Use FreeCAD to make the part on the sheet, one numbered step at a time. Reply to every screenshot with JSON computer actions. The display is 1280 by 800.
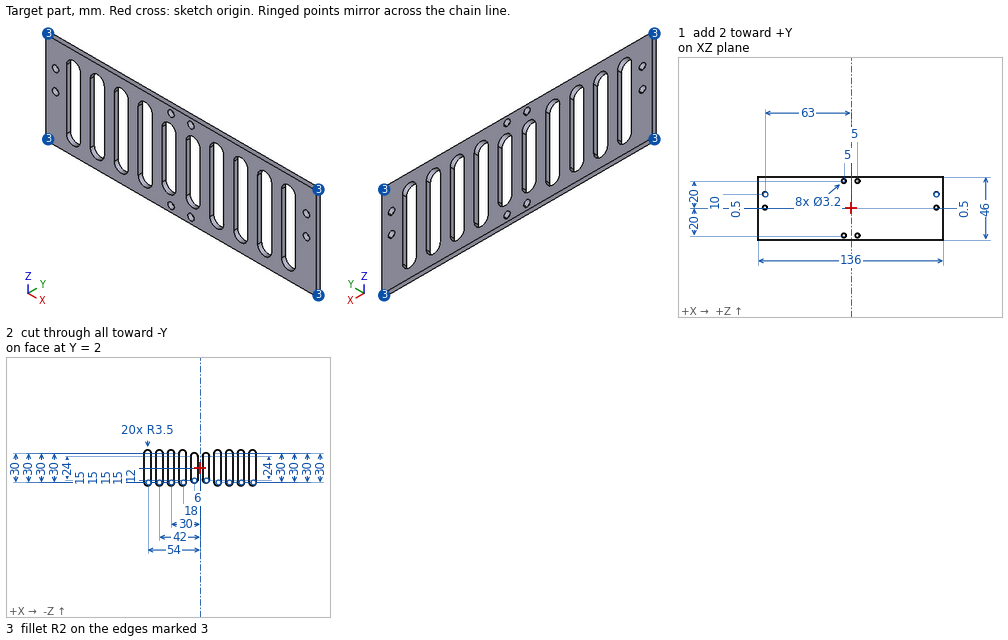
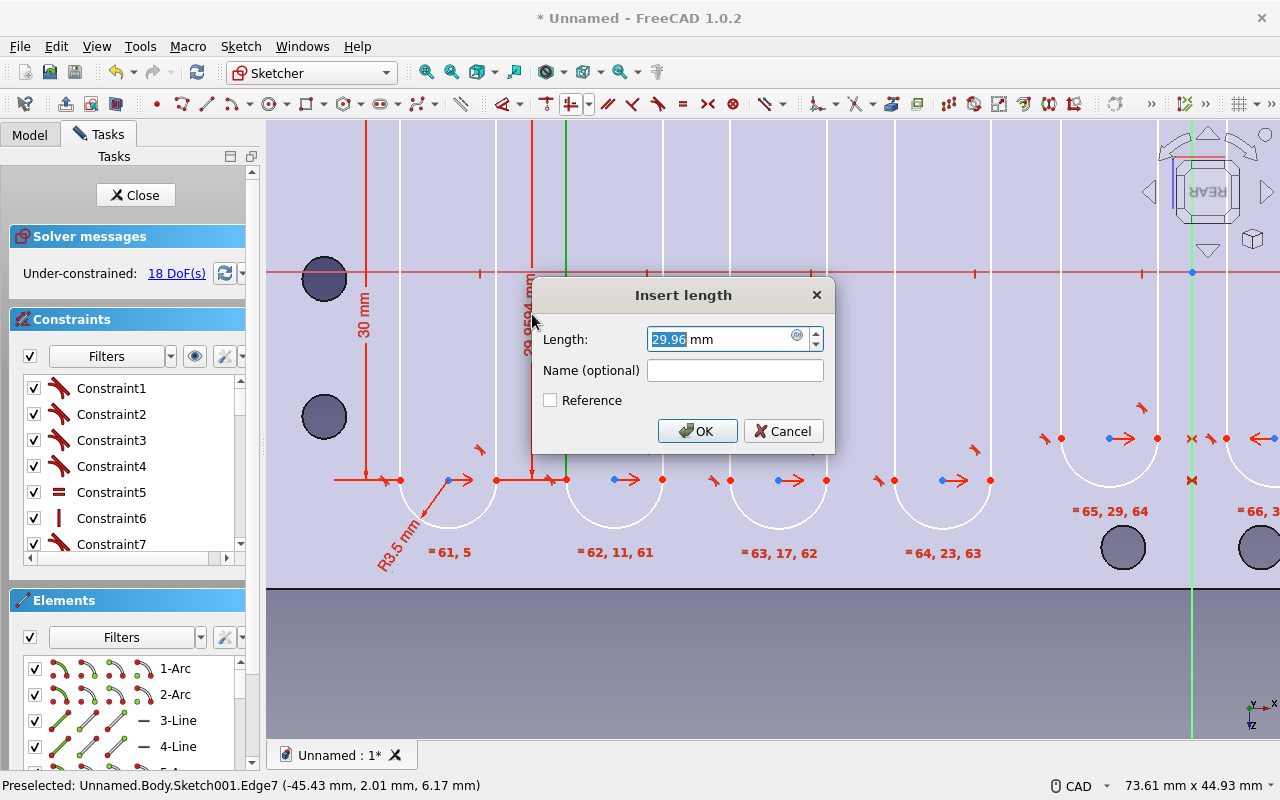
{"action": "type", "text": "30"}
{"action": "key", "text": "Return"}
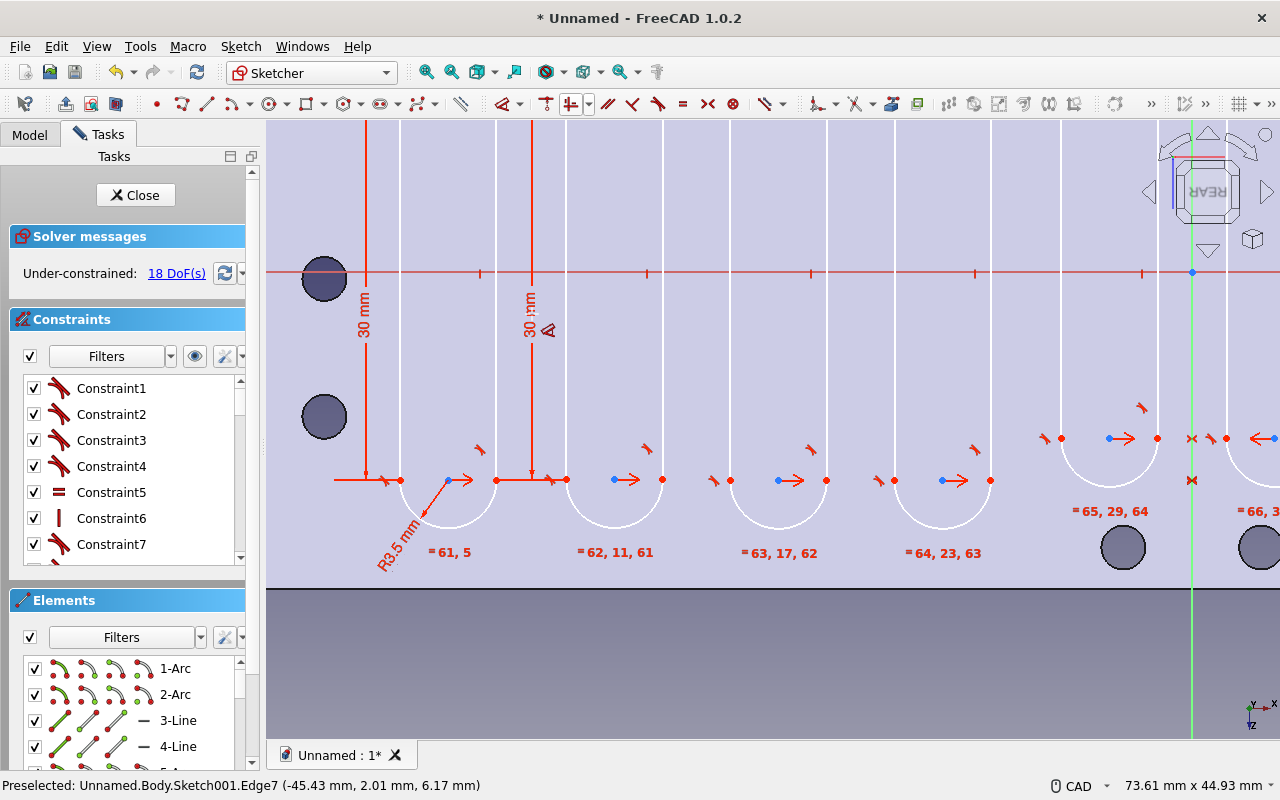
{"action": "left_click", "coordinate": [730, 356]}
{"action": "left_click", "coordinate": [696, 314]}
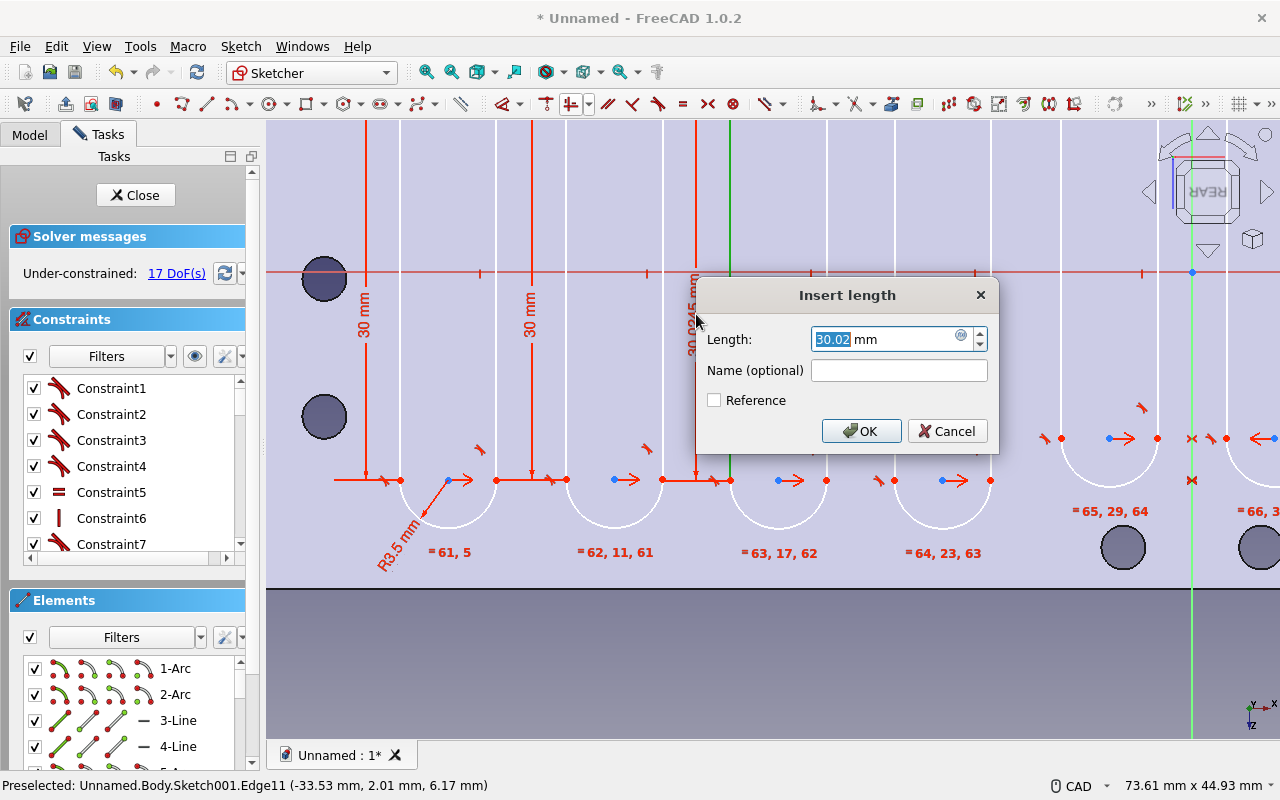
{"action": "type", "text": "30"}
{"action": "key", "text": "Return"}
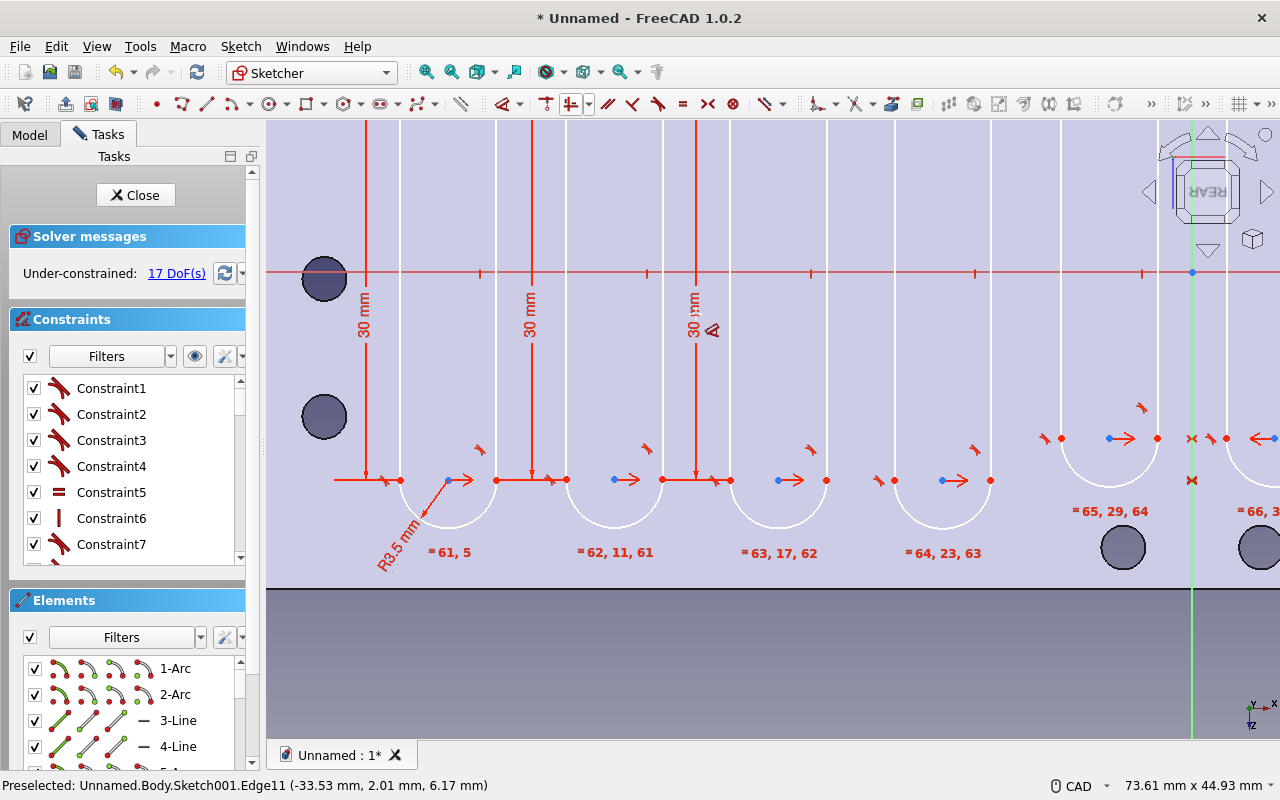
{"action": "left_click", "coordinate": [895, 356]}
{"action": "left_click", "coordinate": [861, 314]}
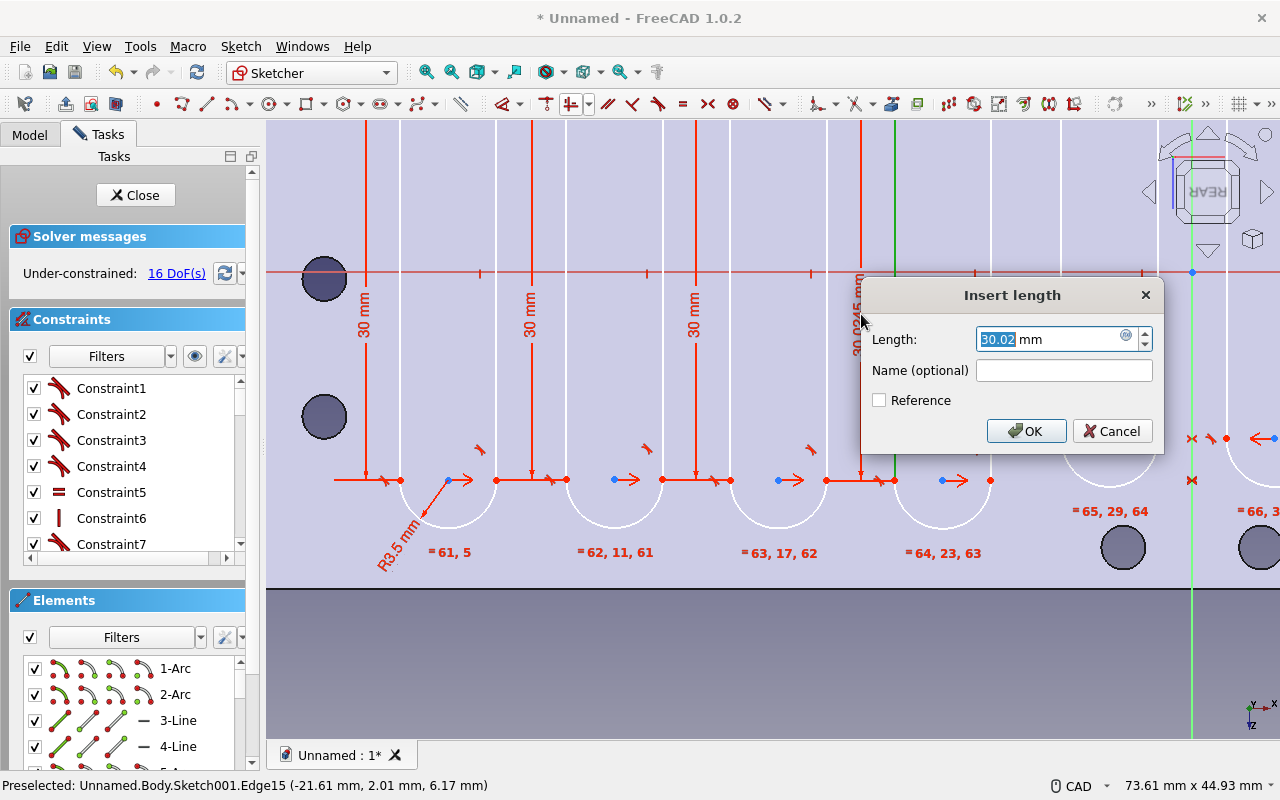
{"action": "type", "text": "30"}
{"action": "key", "text": "Return"}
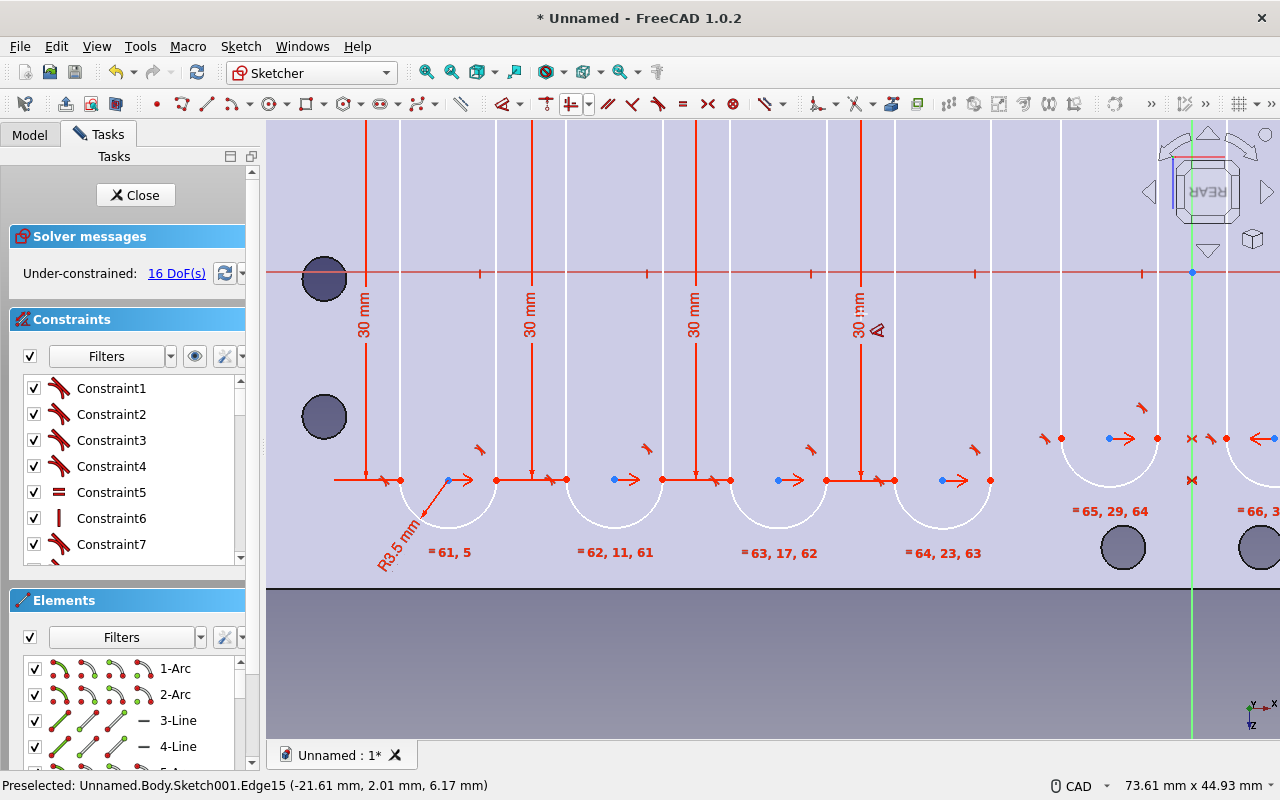
{"action": "left_click", "coordinate": [1061, 340]}
{"action": "left_click", "coordinate": [1027, 293]}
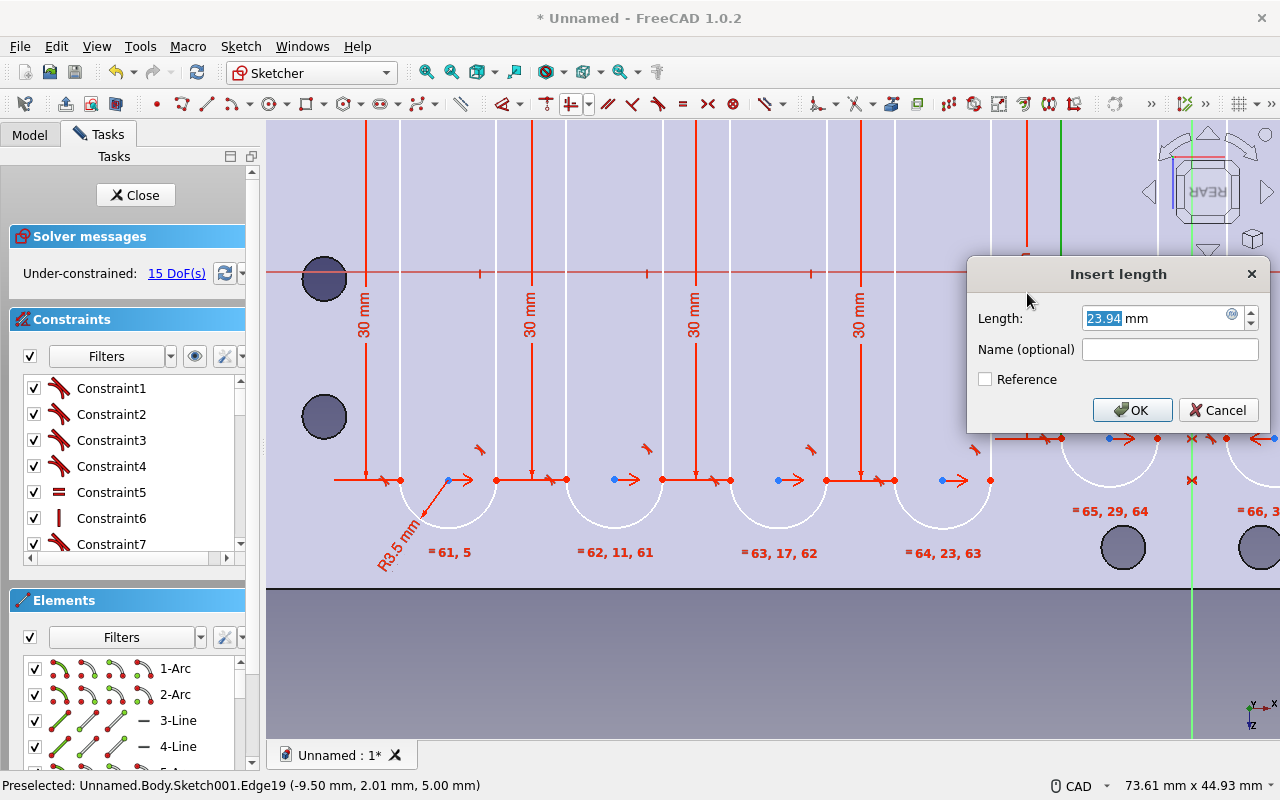
{"action": "type", "text": "24"}
{"action": "key", "text": "Return"}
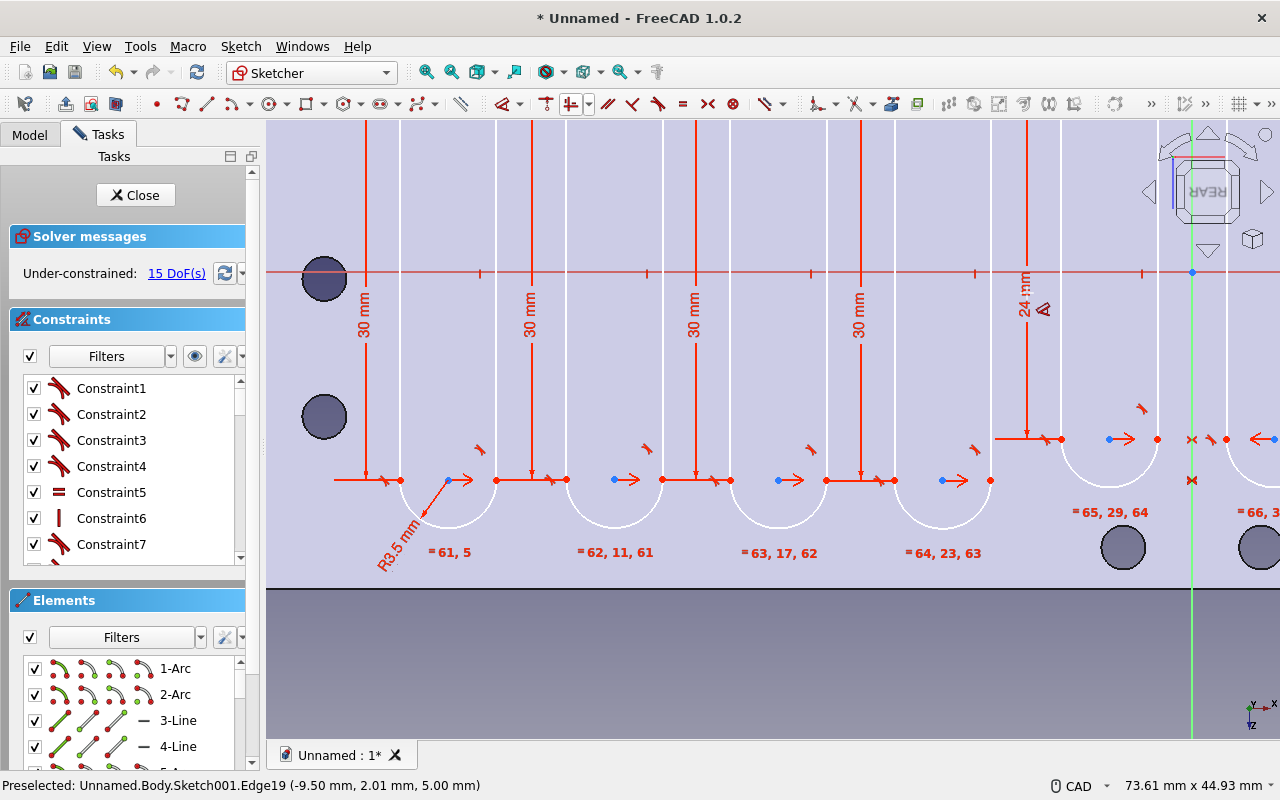
{"action": "scroll", "coordinate": [421, 521], "scroll_direction": "down", "scroll_amount": 5}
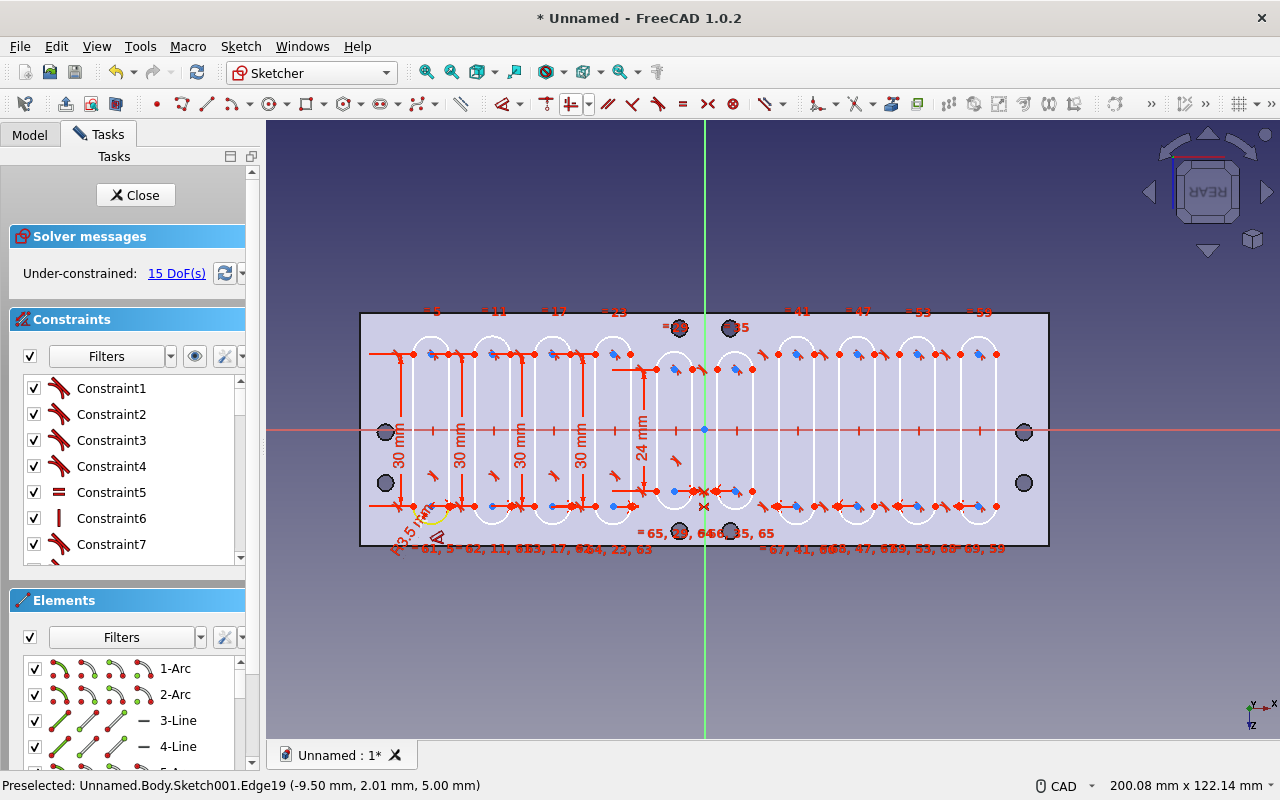
{"action": "left_click", "coordinate": [717, 455]}
{"action": "left_click", "coordinate": [799, 403]}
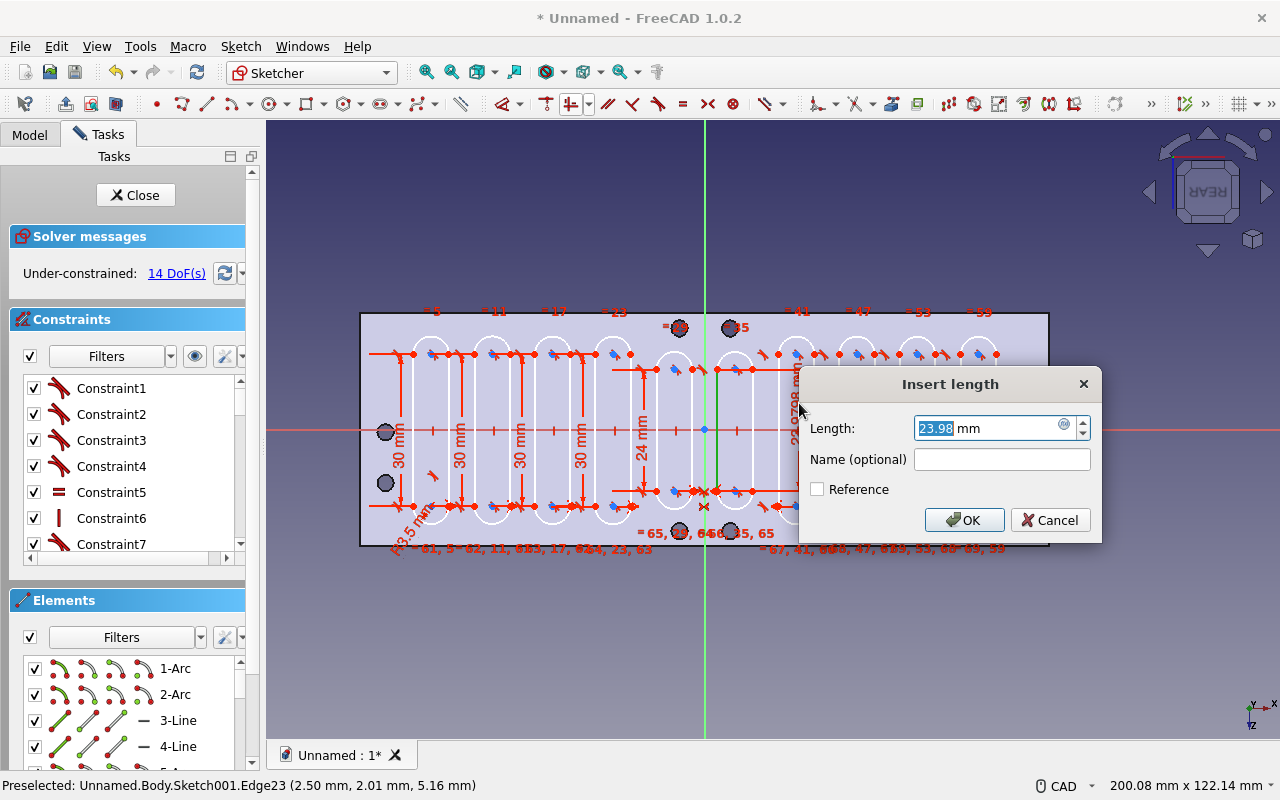
{"action": "type", "text": "24"}
{"action": "key", "text": "Return"}